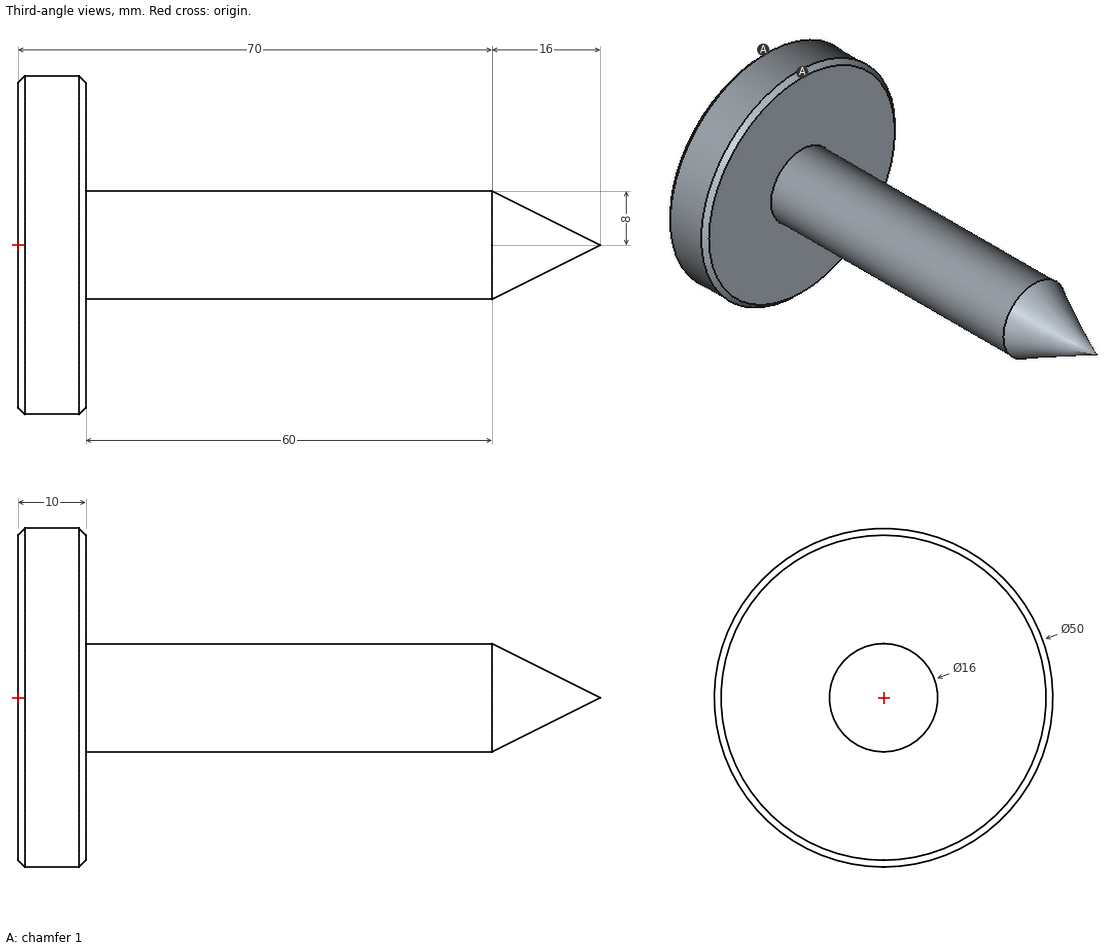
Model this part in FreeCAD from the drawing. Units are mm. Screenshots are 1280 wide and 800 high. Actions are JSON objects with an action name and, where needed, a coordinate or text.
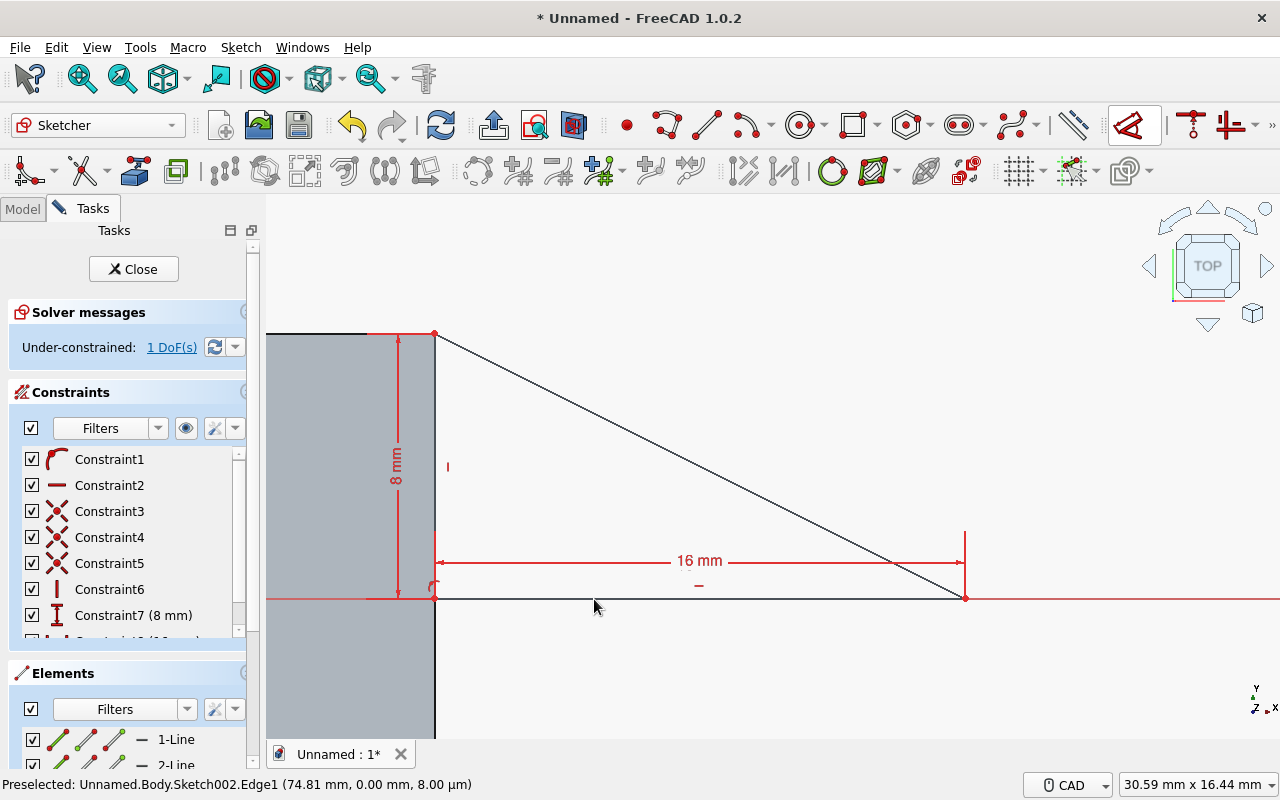
{"action": "left_click", "coordinate": [435, 599]}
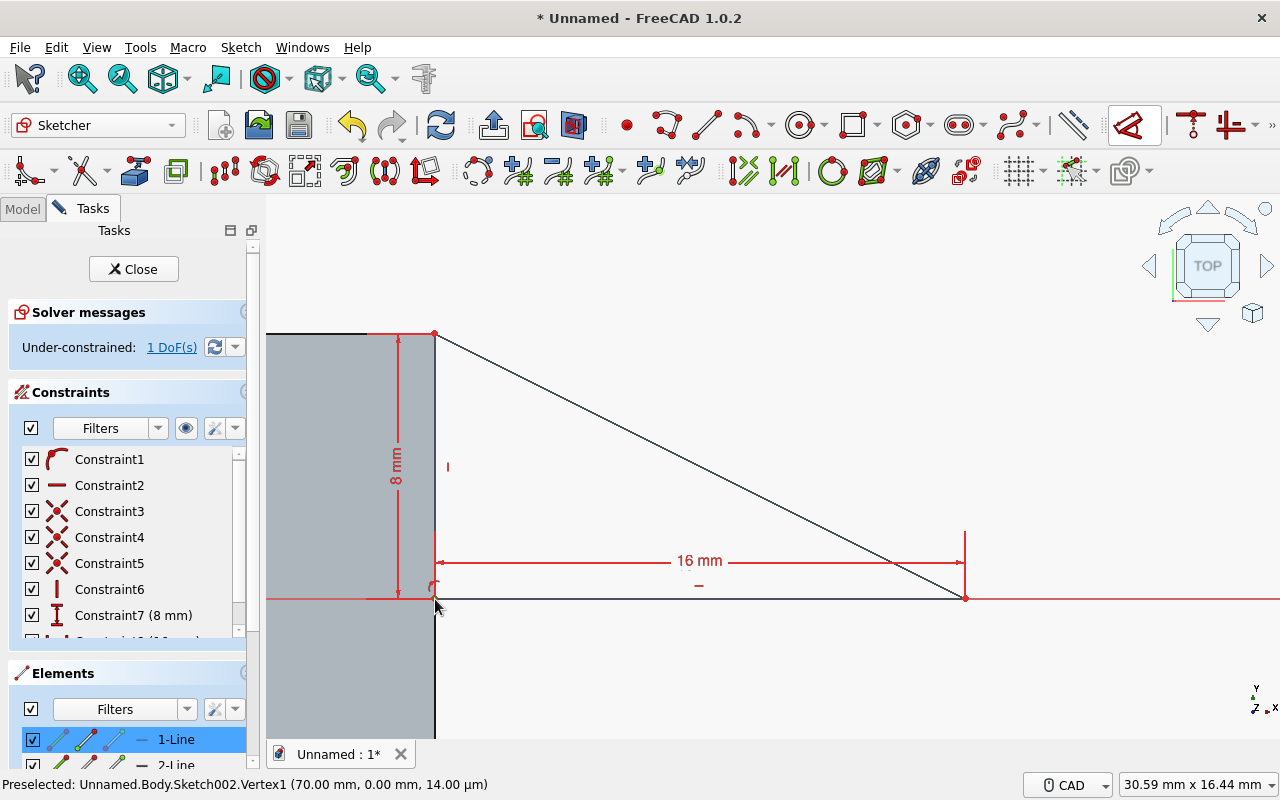
{"action": "key", "text": "l"}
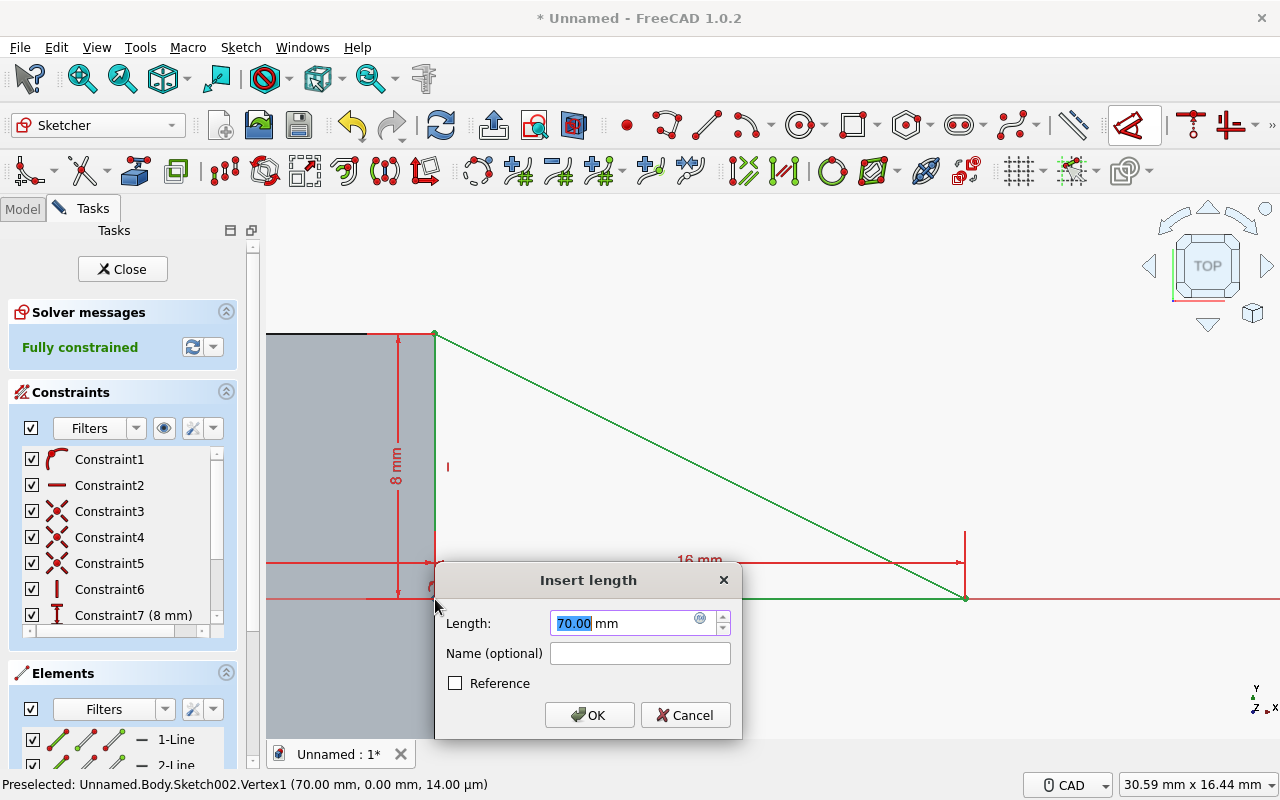
{"action": "type", "text": "70"}
{"action": "key", "text": "Return"}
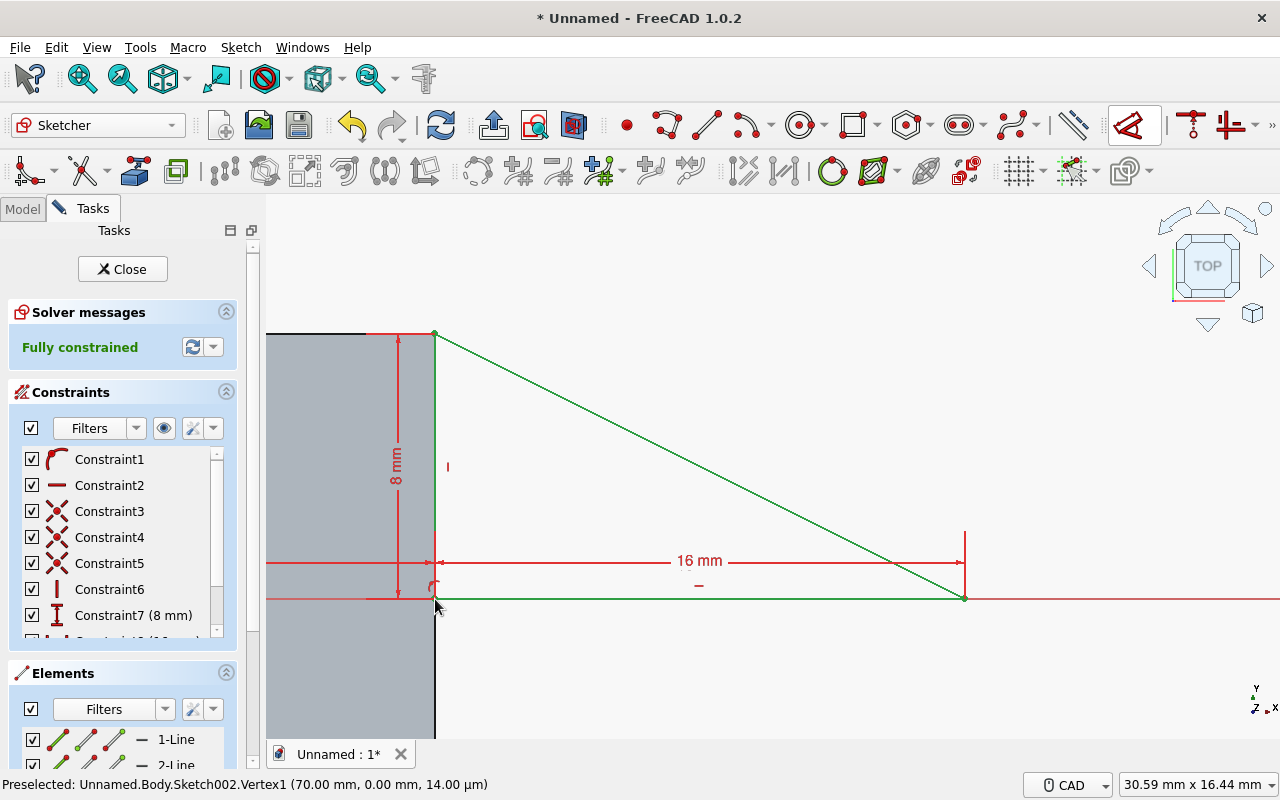
{"action": "left_click", "coordinate": [123, 269]}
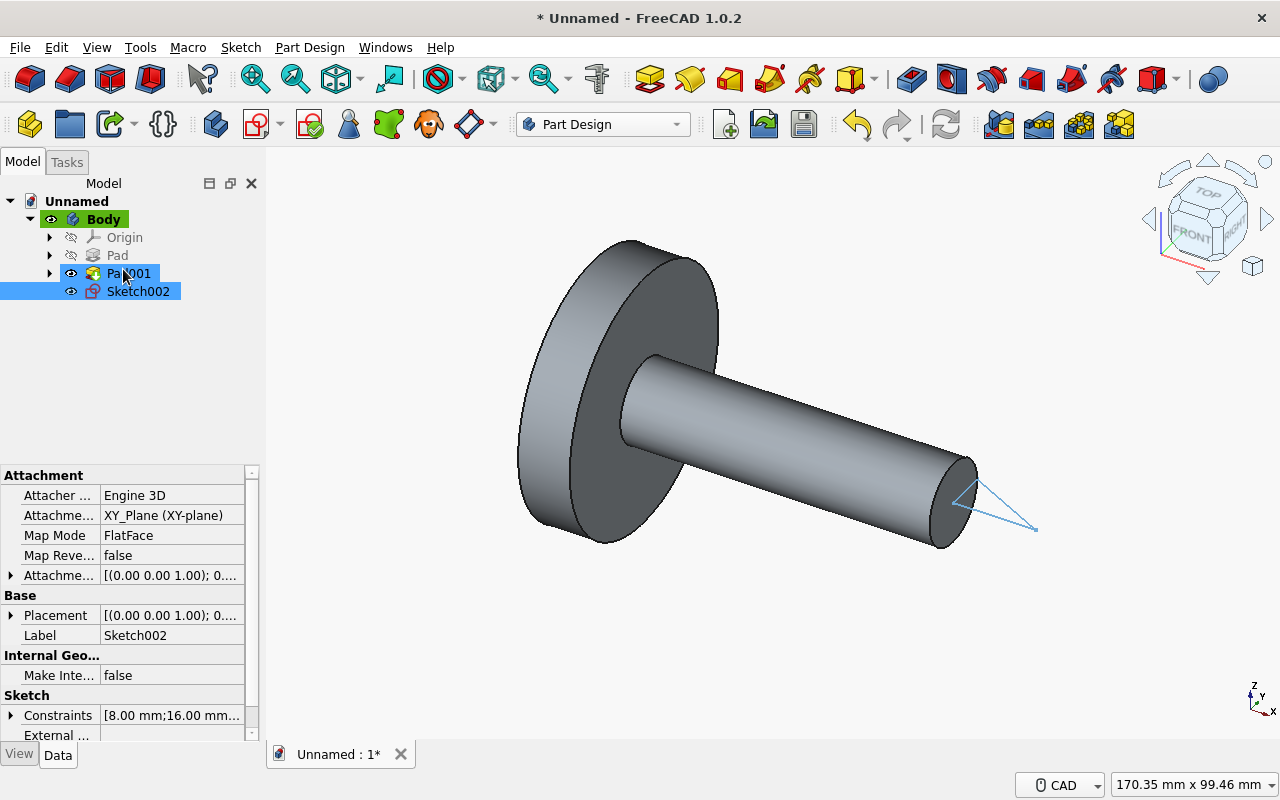
{"action": "left_click", "coordinate": [690, 80]}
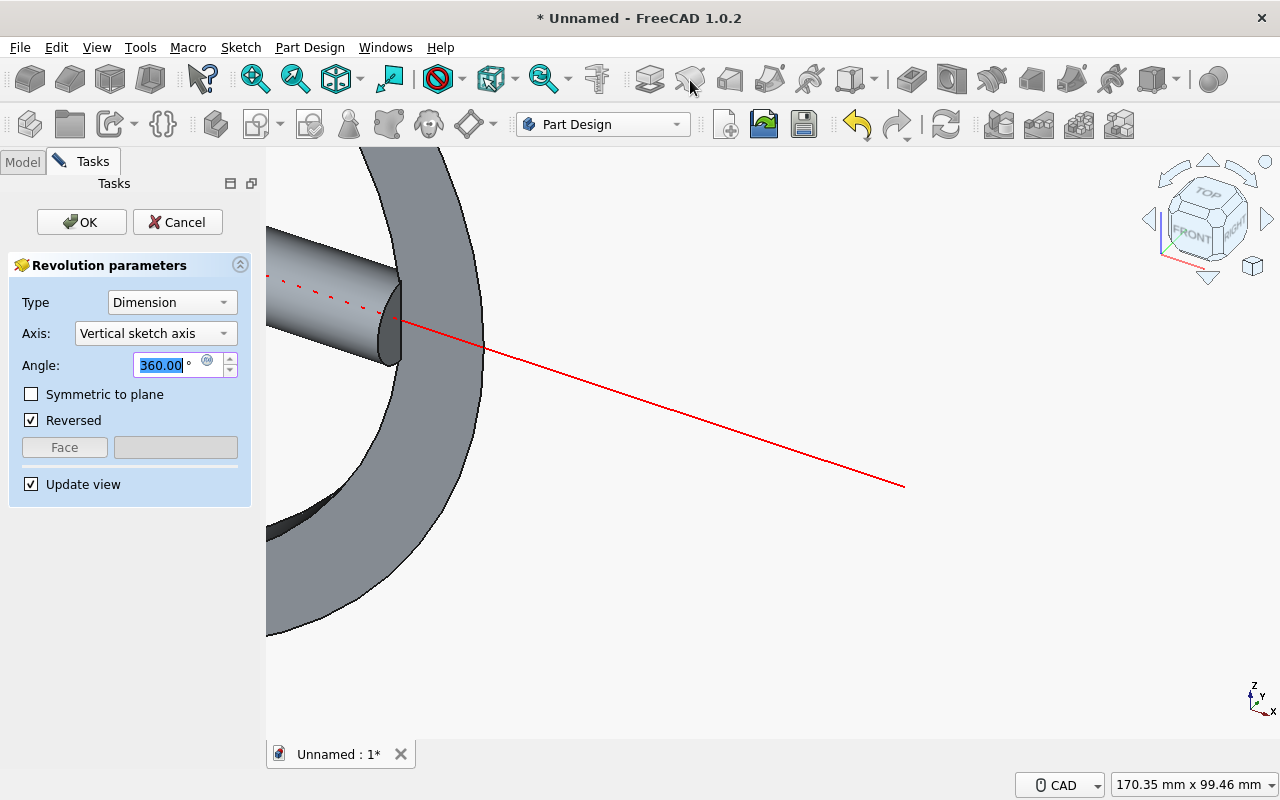
{"action": "left_click", "coordinate": [156, 334]}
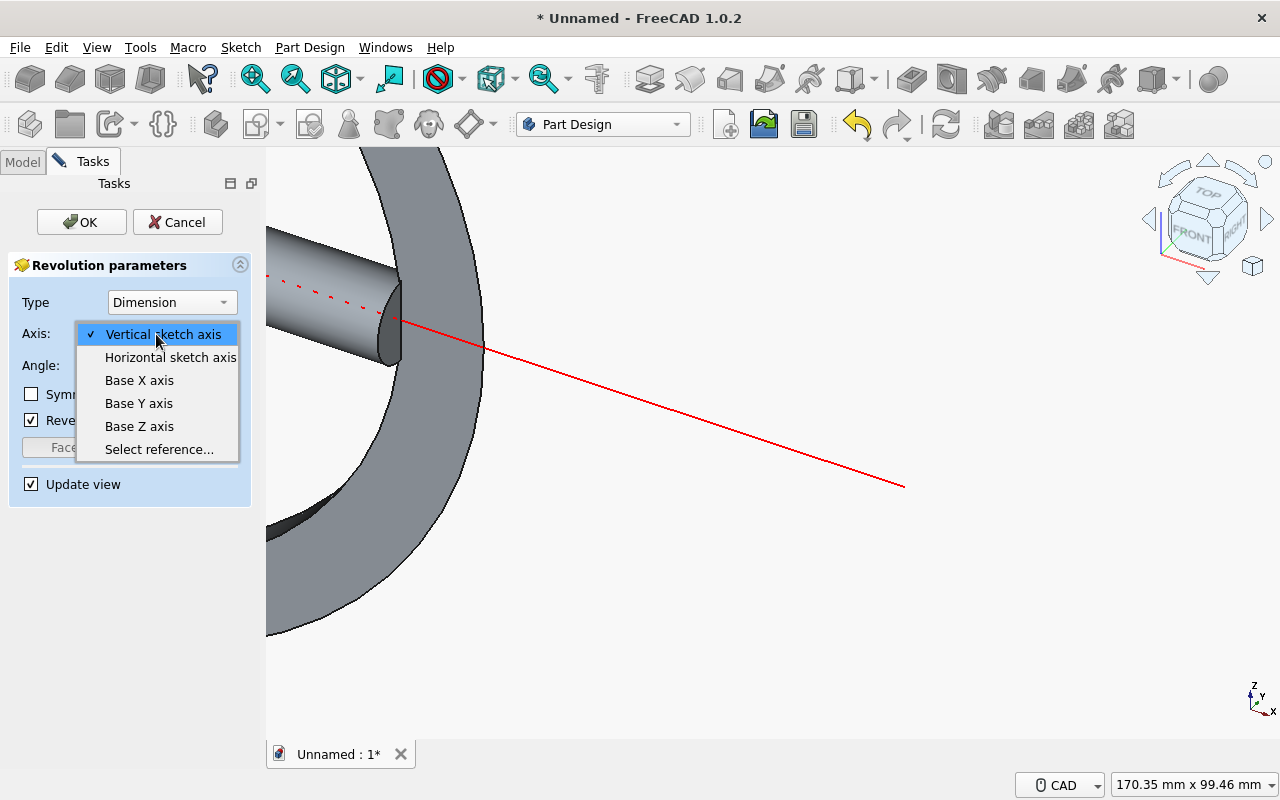
{"action": "left_click", "coordinate": [156, 358]}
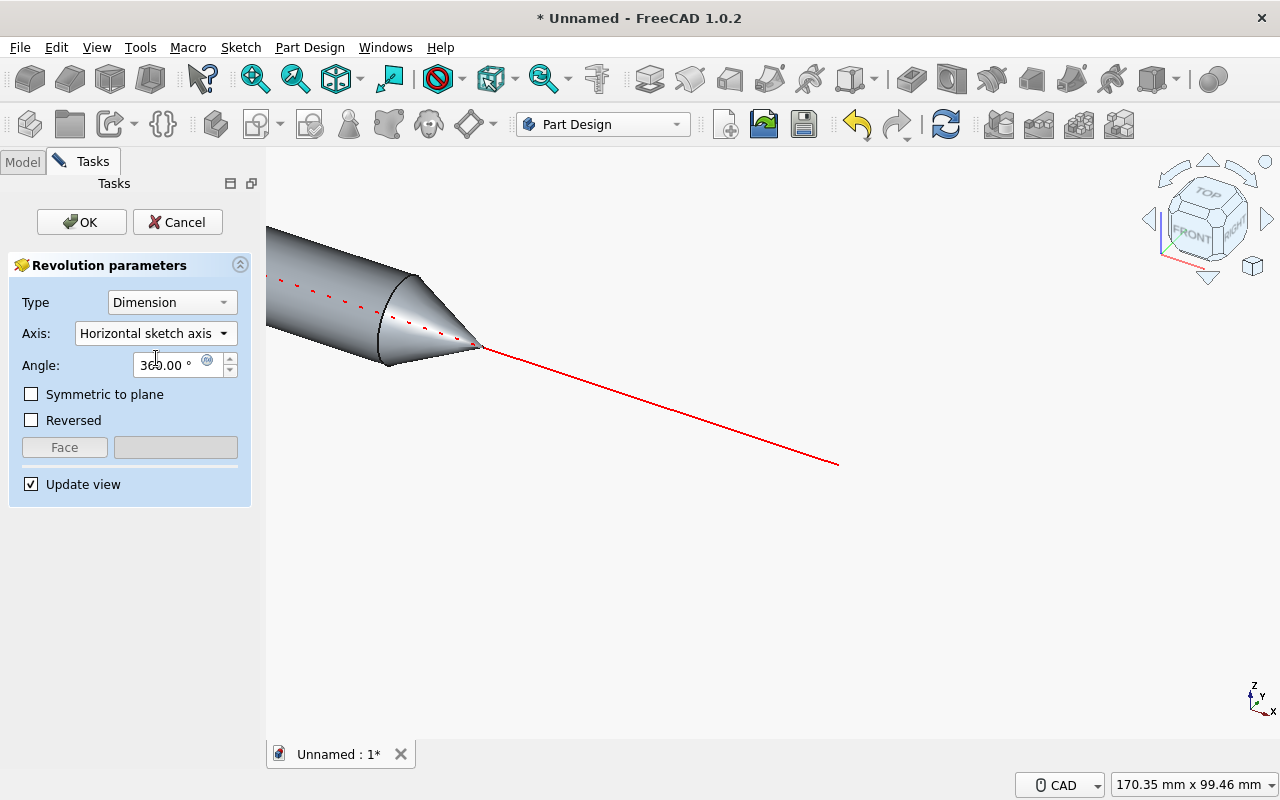
{"action": "left_click", "coordinate": [82, 222]}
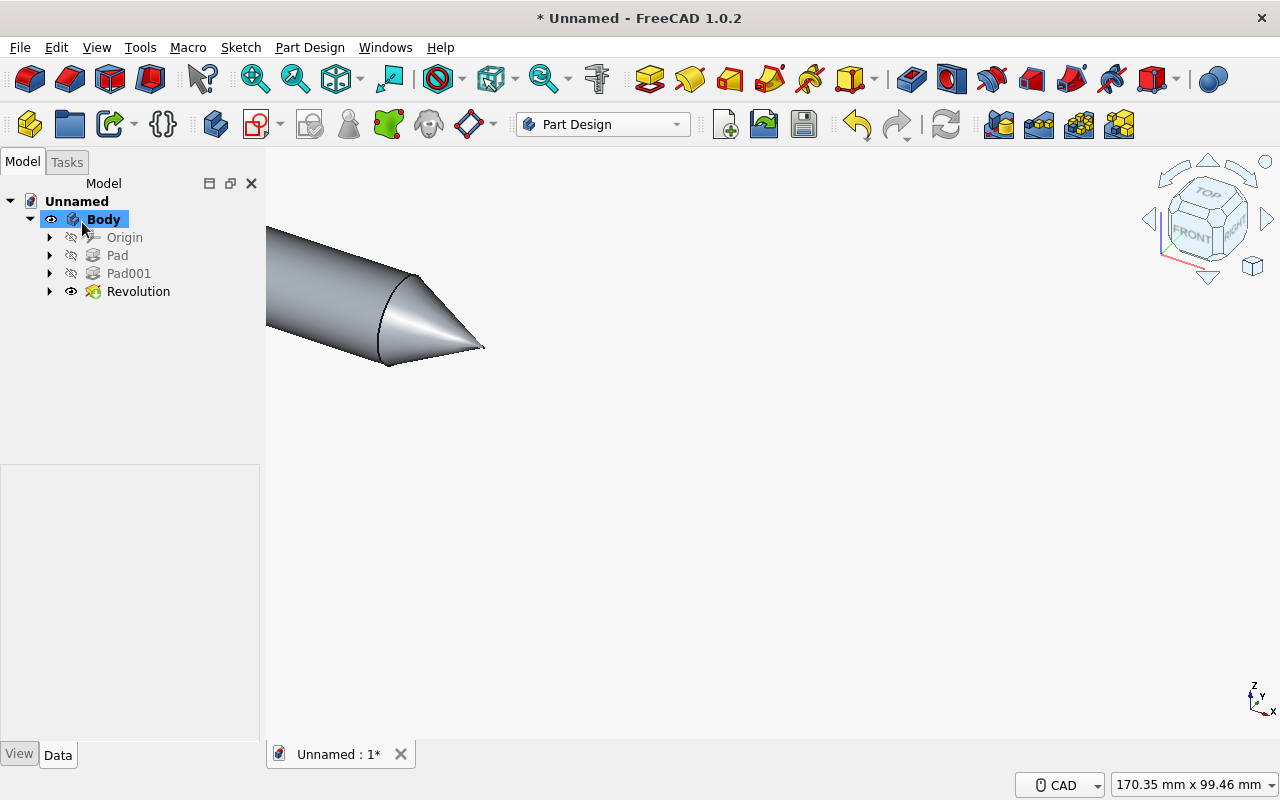
{"action": "key", "text": "v f"}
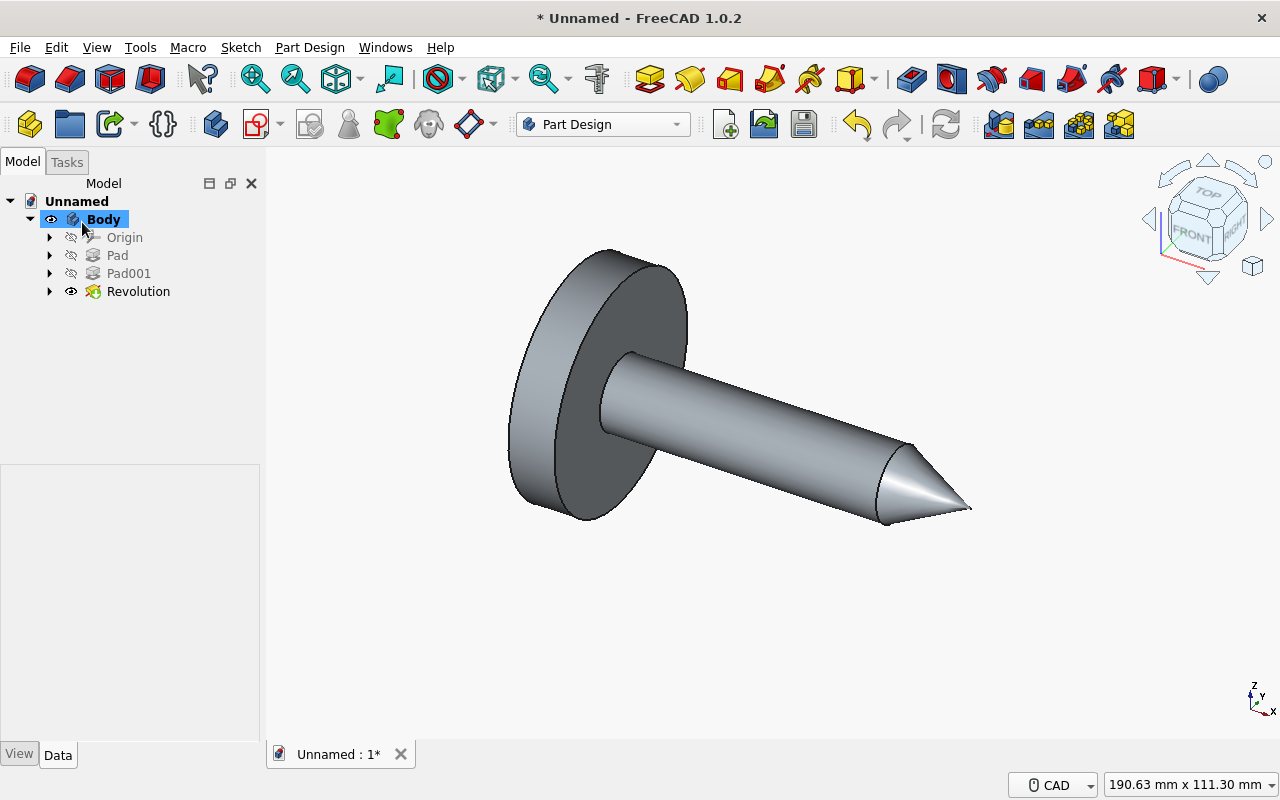
{"action": "left_click", "coordinate": [554, 458]}